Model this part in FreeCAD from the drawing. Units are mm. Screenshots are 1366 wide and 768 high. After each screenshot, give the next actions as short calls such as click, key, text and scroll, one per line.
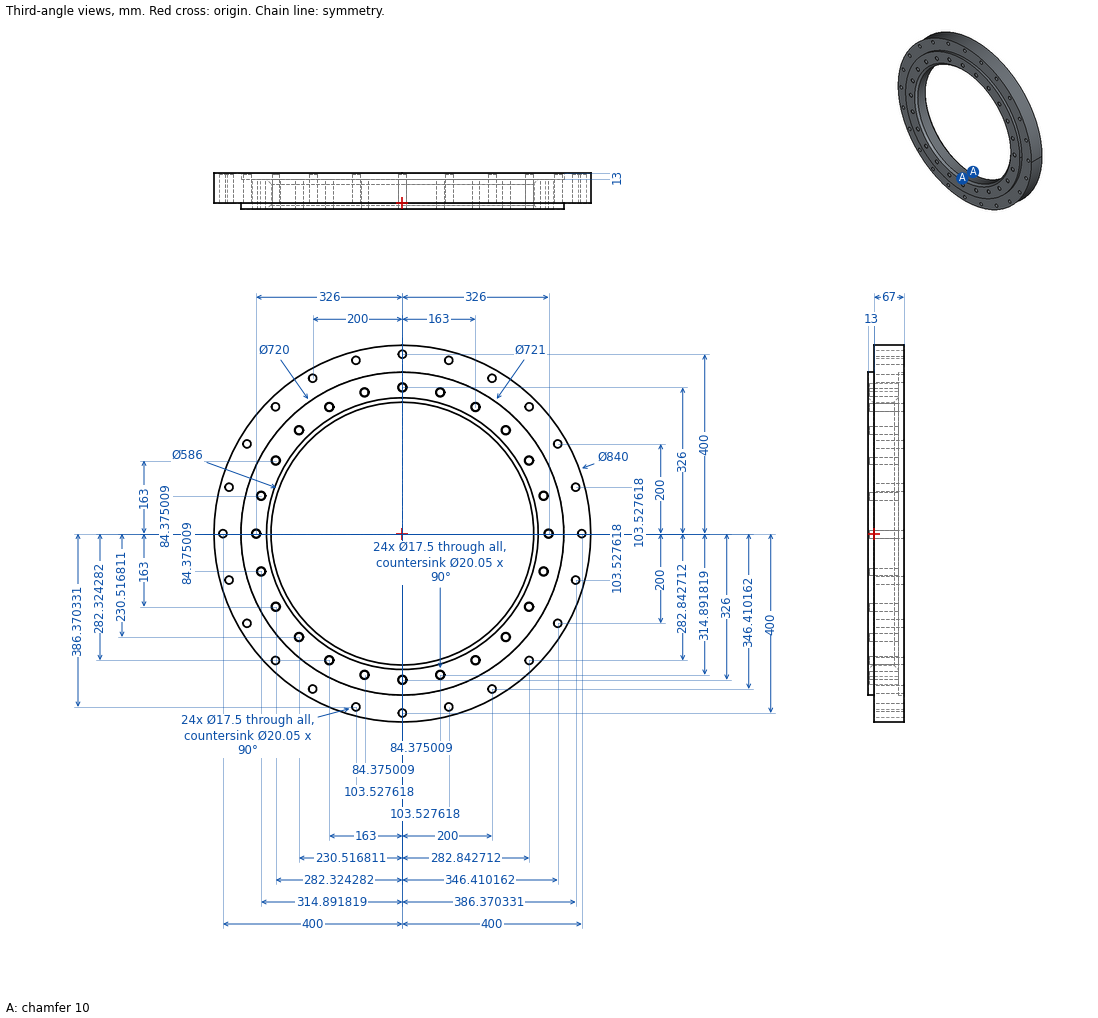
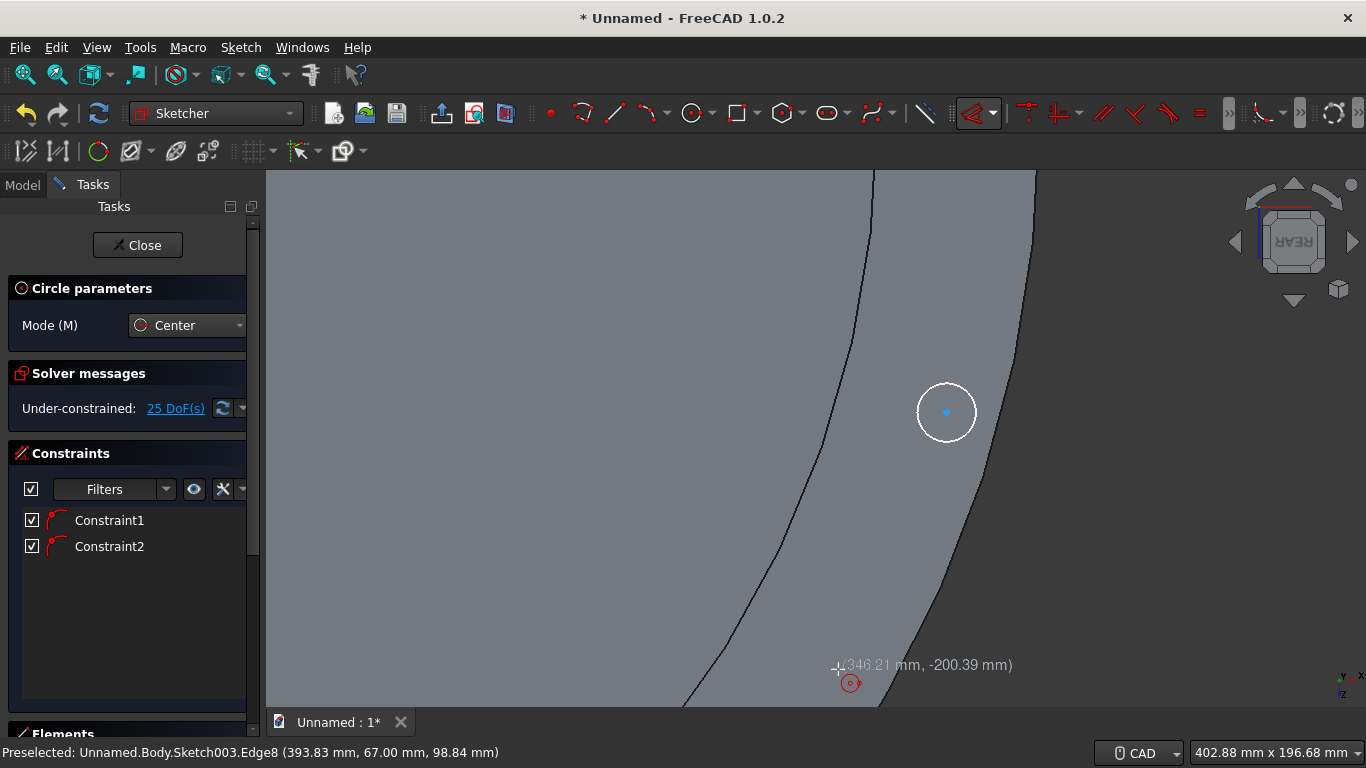
scroll(917, 501, down, 9)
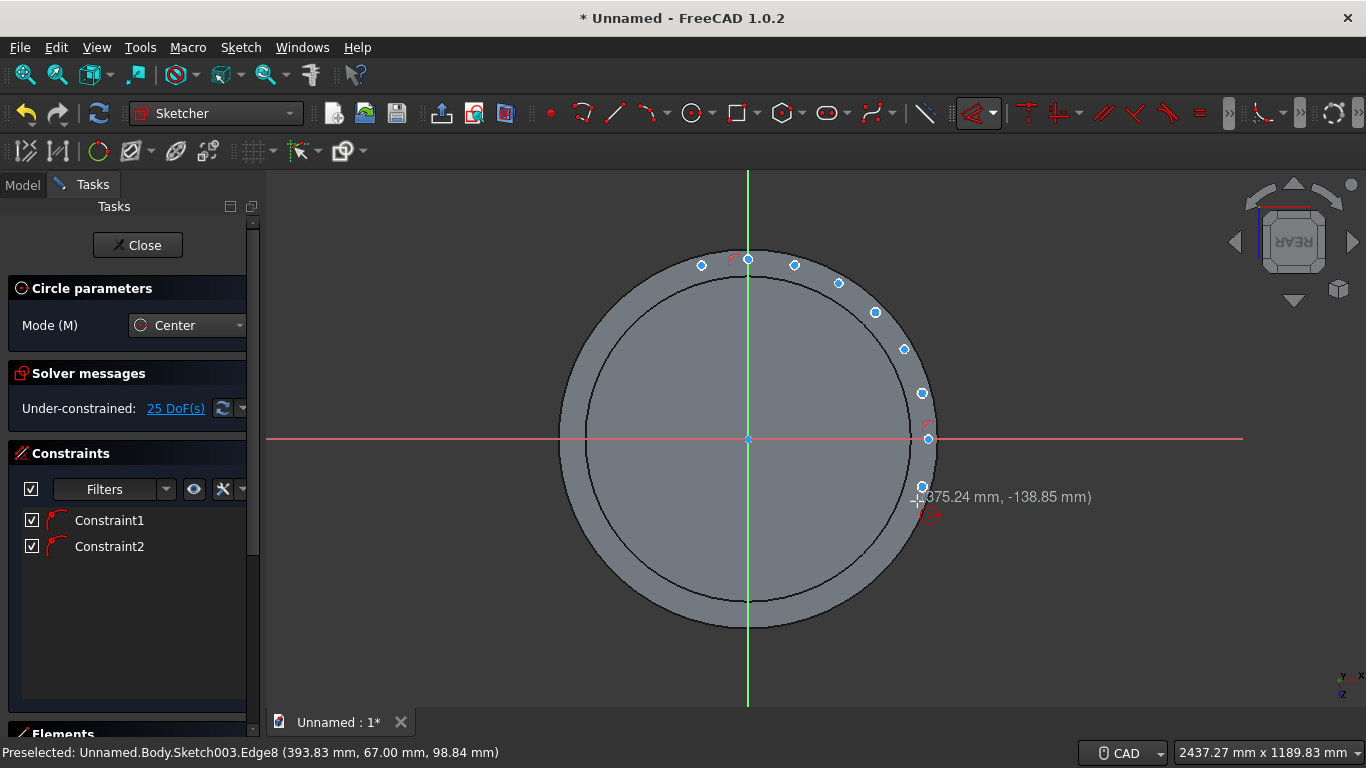
click(904, 529)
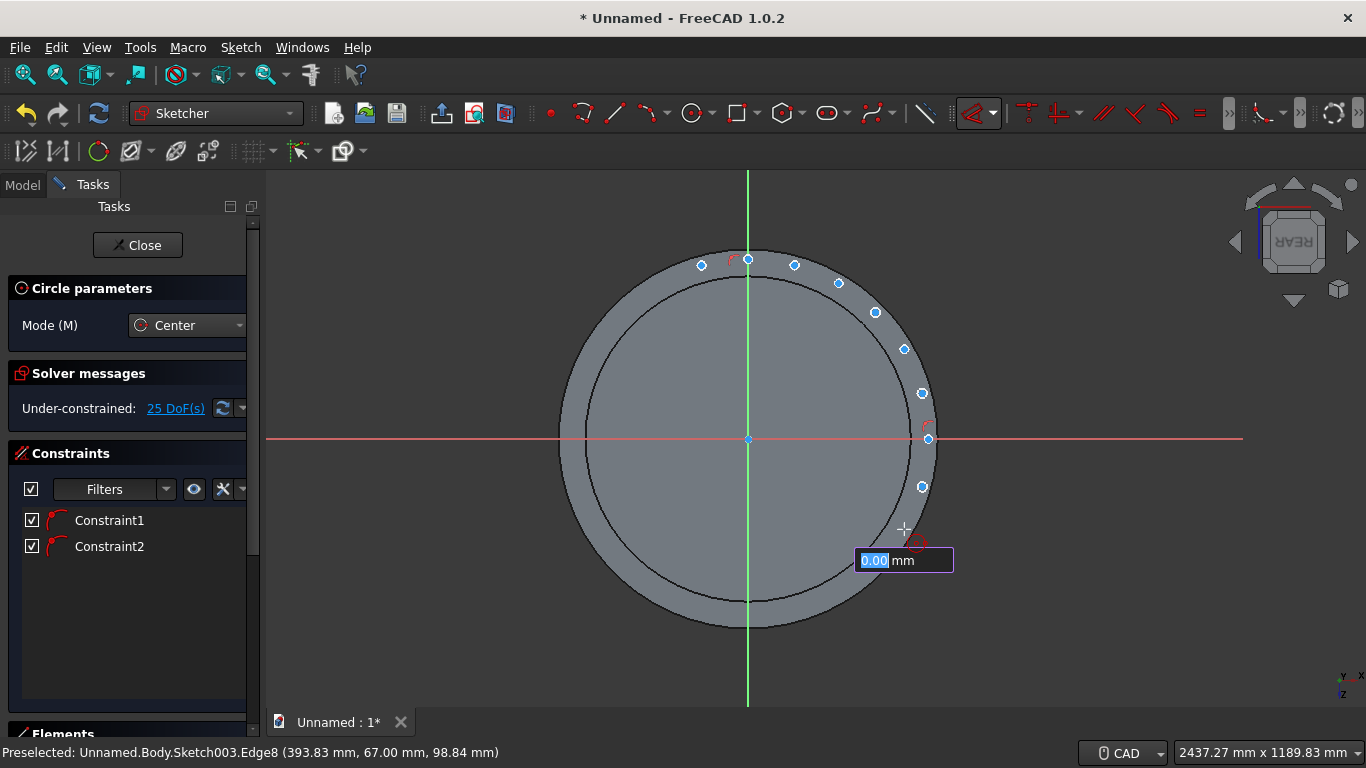
scroll(907, 526, up, 7)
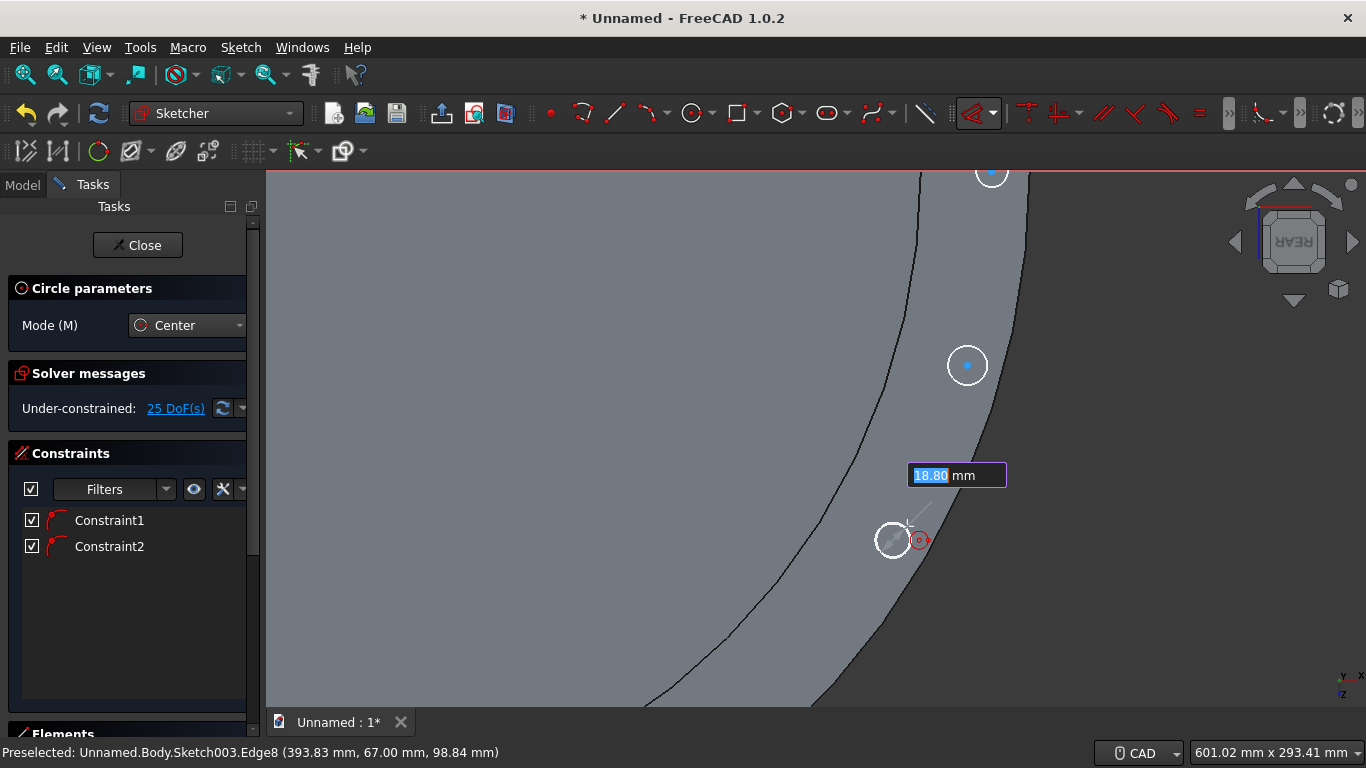
click(906, 526)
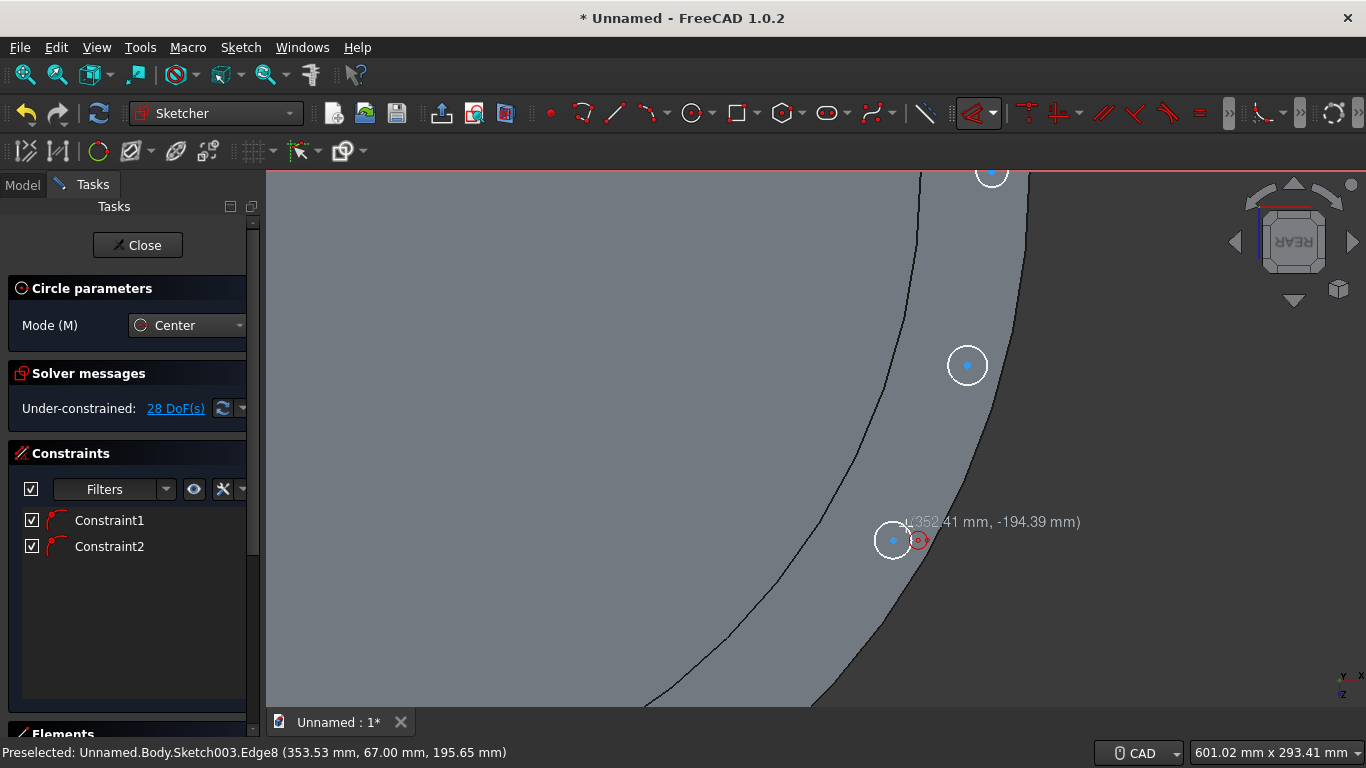
scroll(907, 526, down, 7)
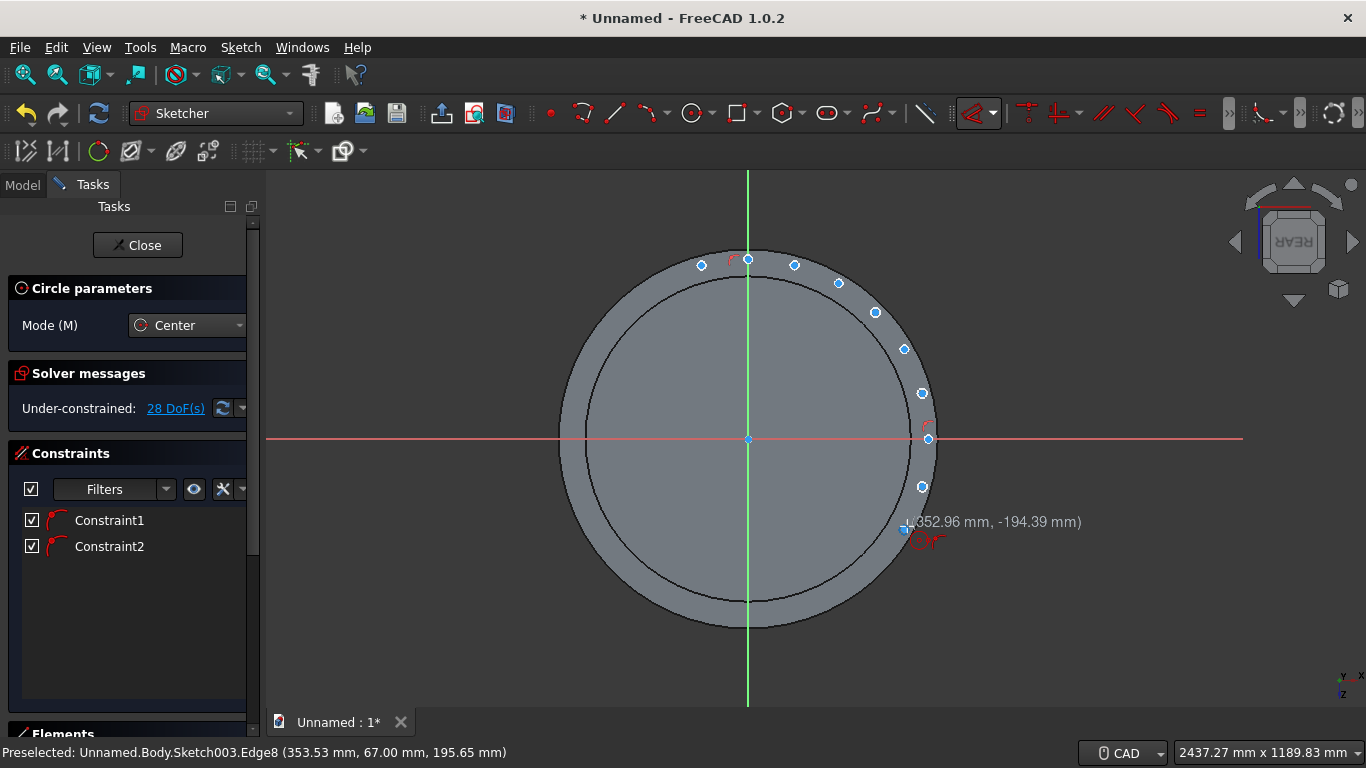
scroll(876, 567, up, 9)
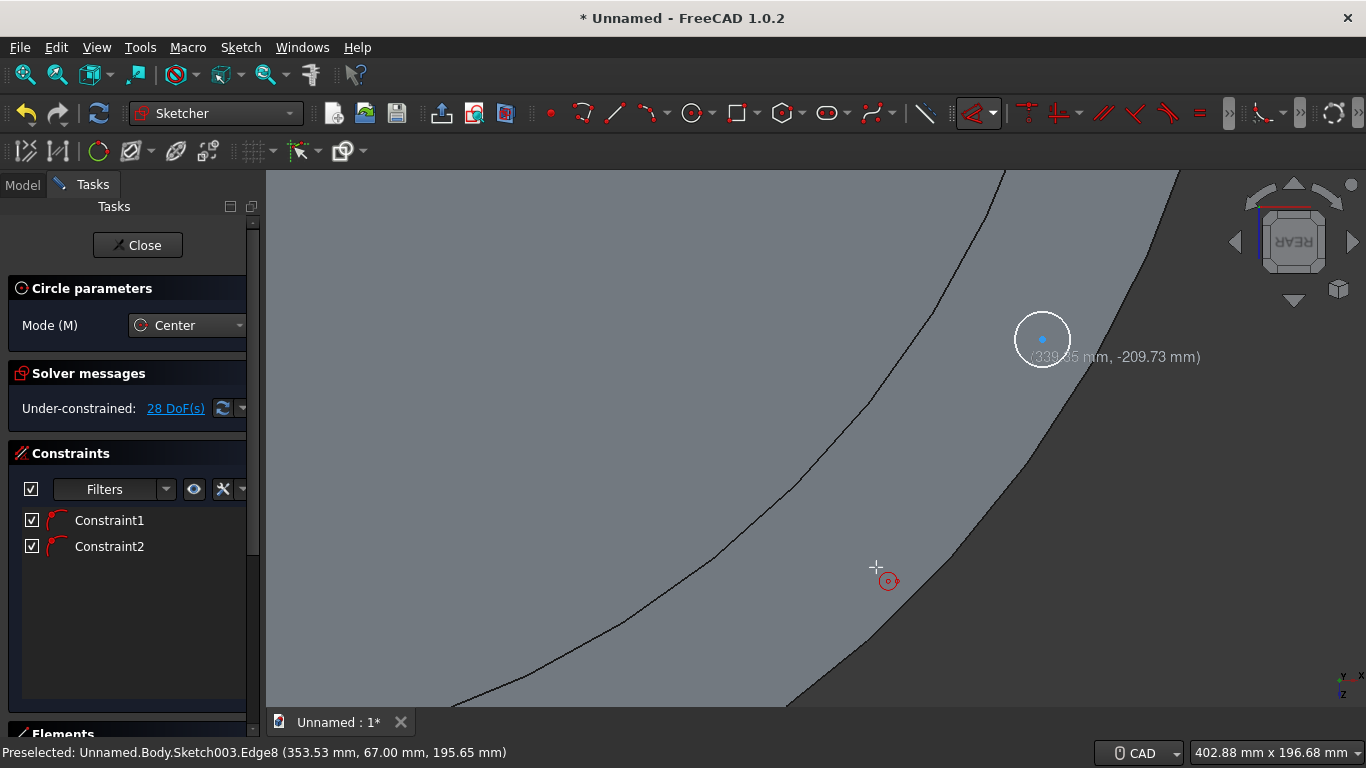
scroll(876, 567, down, 9)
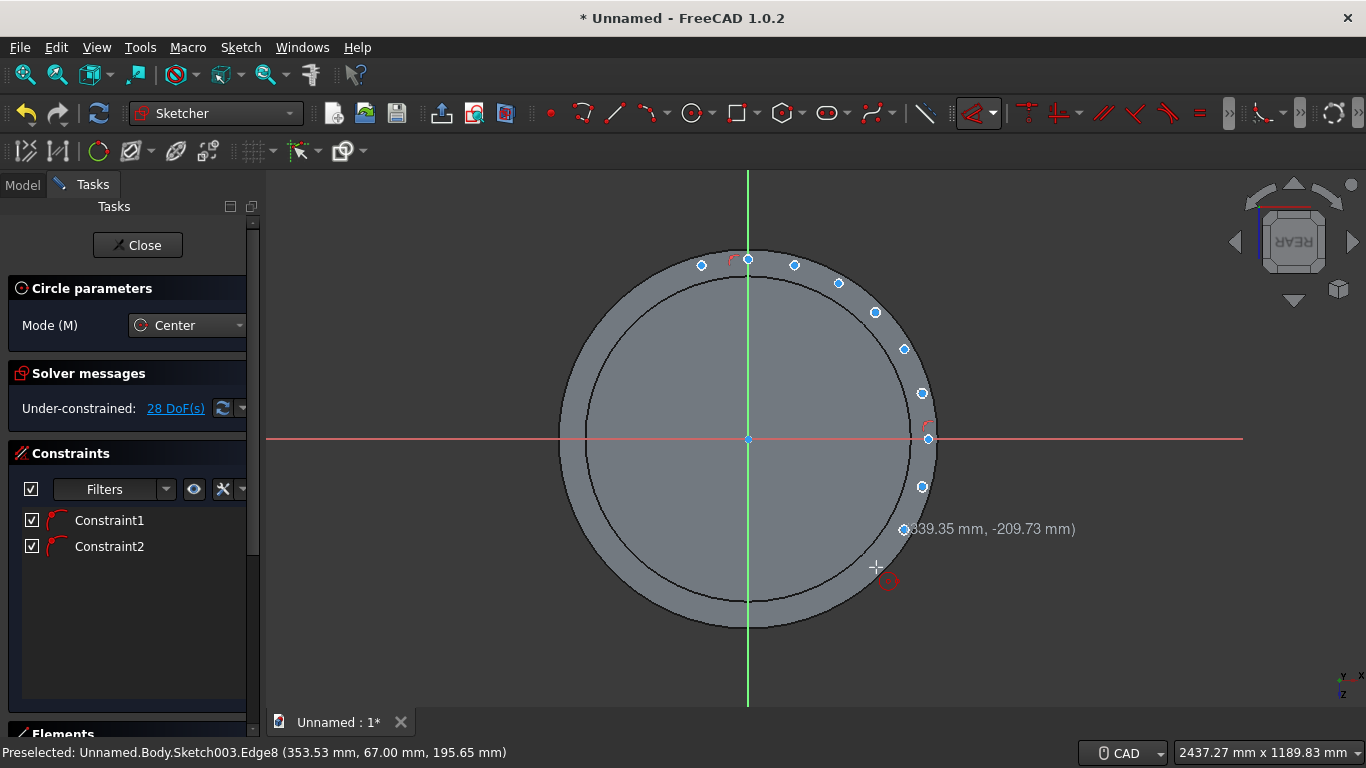
click(876, 567)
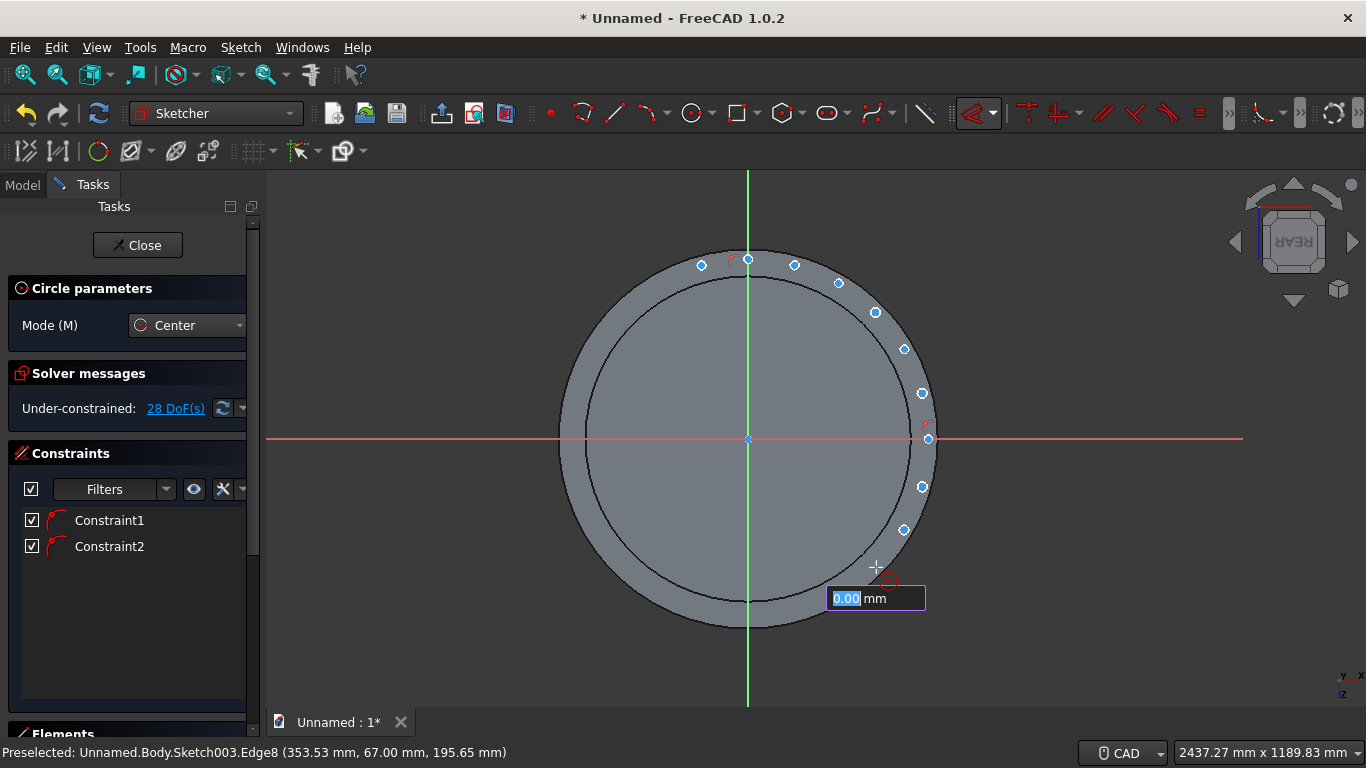
scroll(879, 564, up, 7)